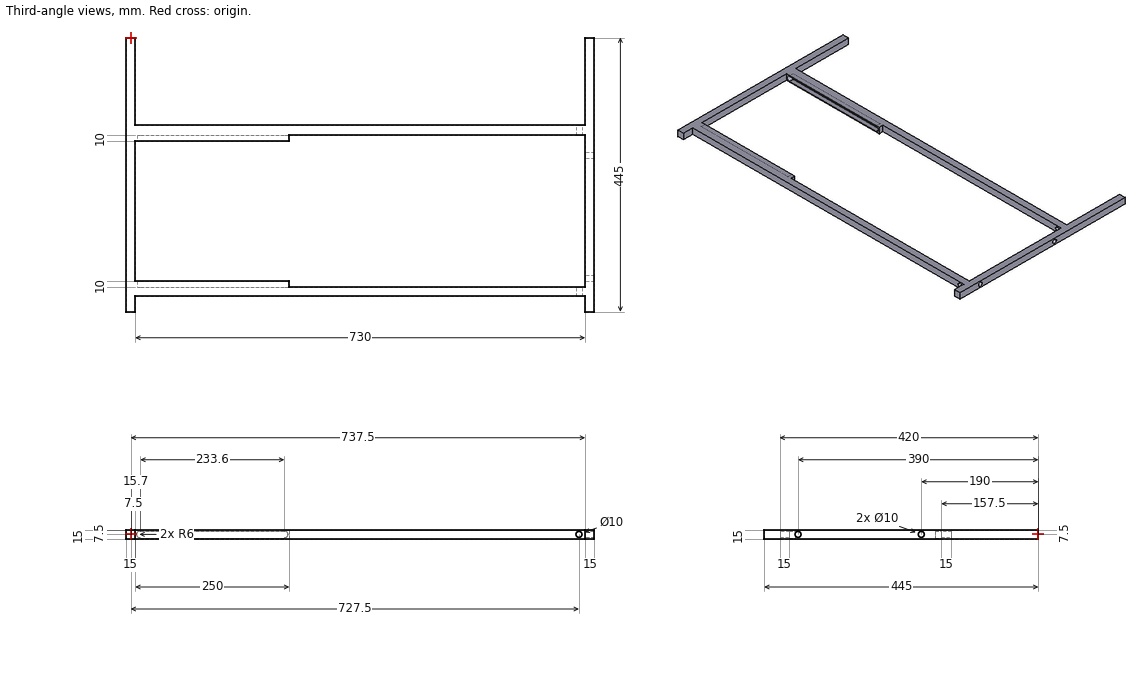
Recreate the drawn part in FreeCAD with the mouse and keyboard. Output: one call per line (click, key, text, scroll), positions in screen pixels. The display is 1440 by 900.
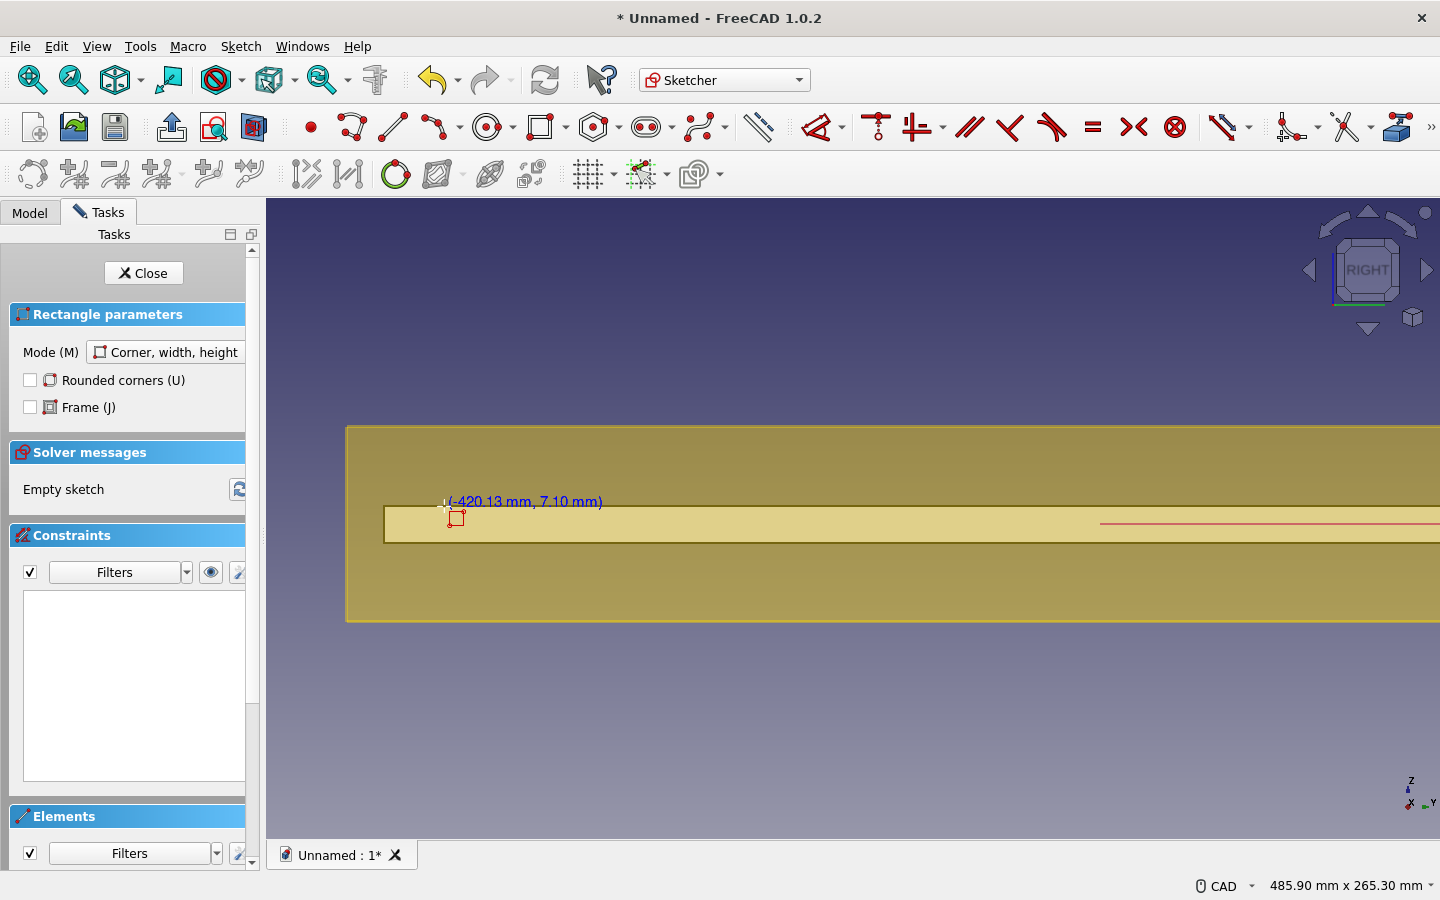
click(444, 506)
click(480, 543)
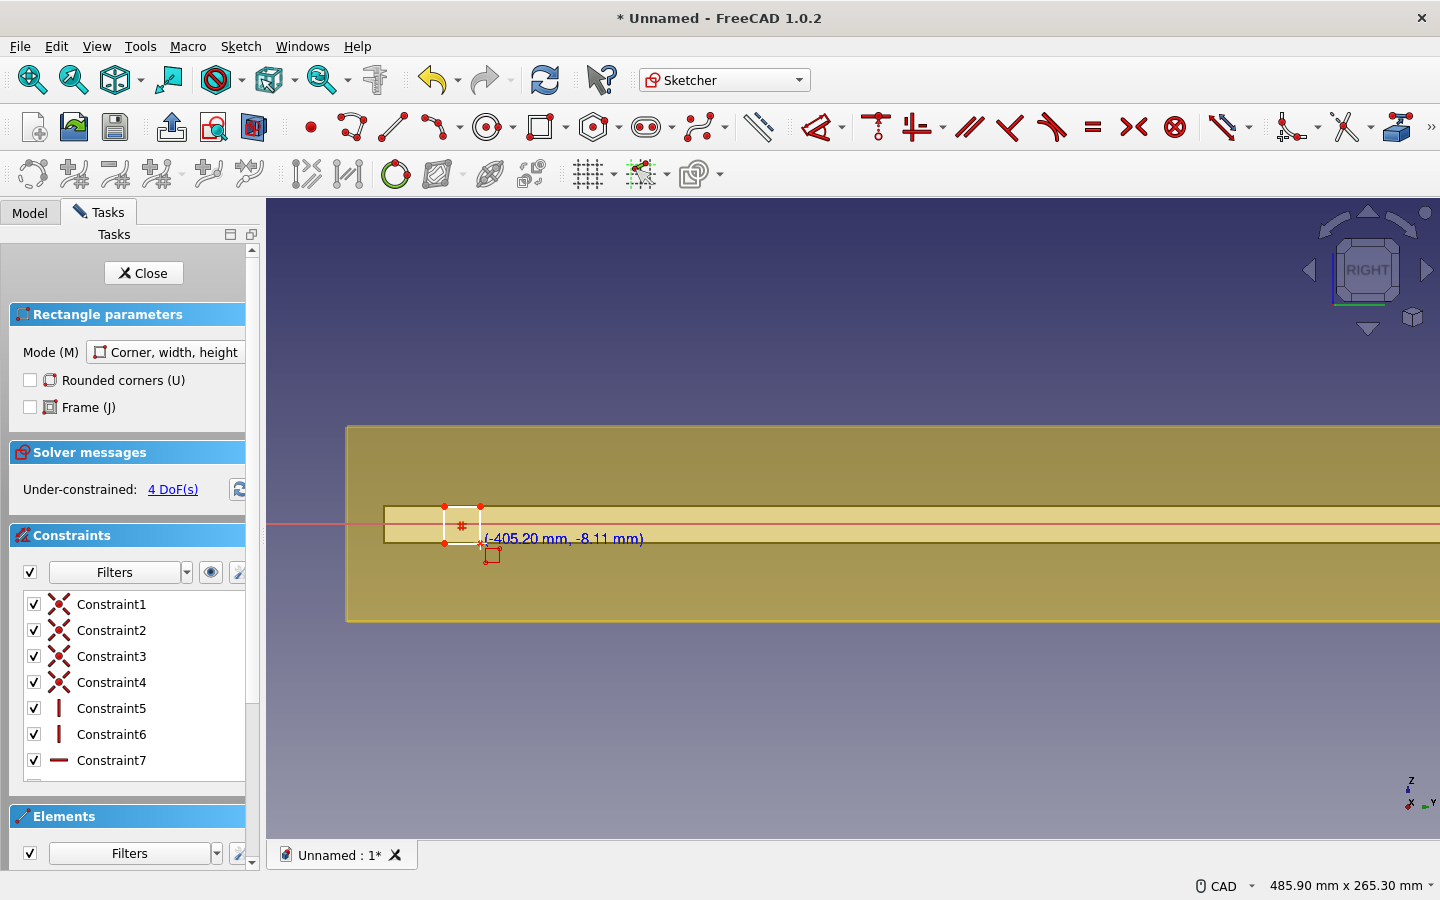
click(1078, 506)
click(1115, 543)
key(Escape)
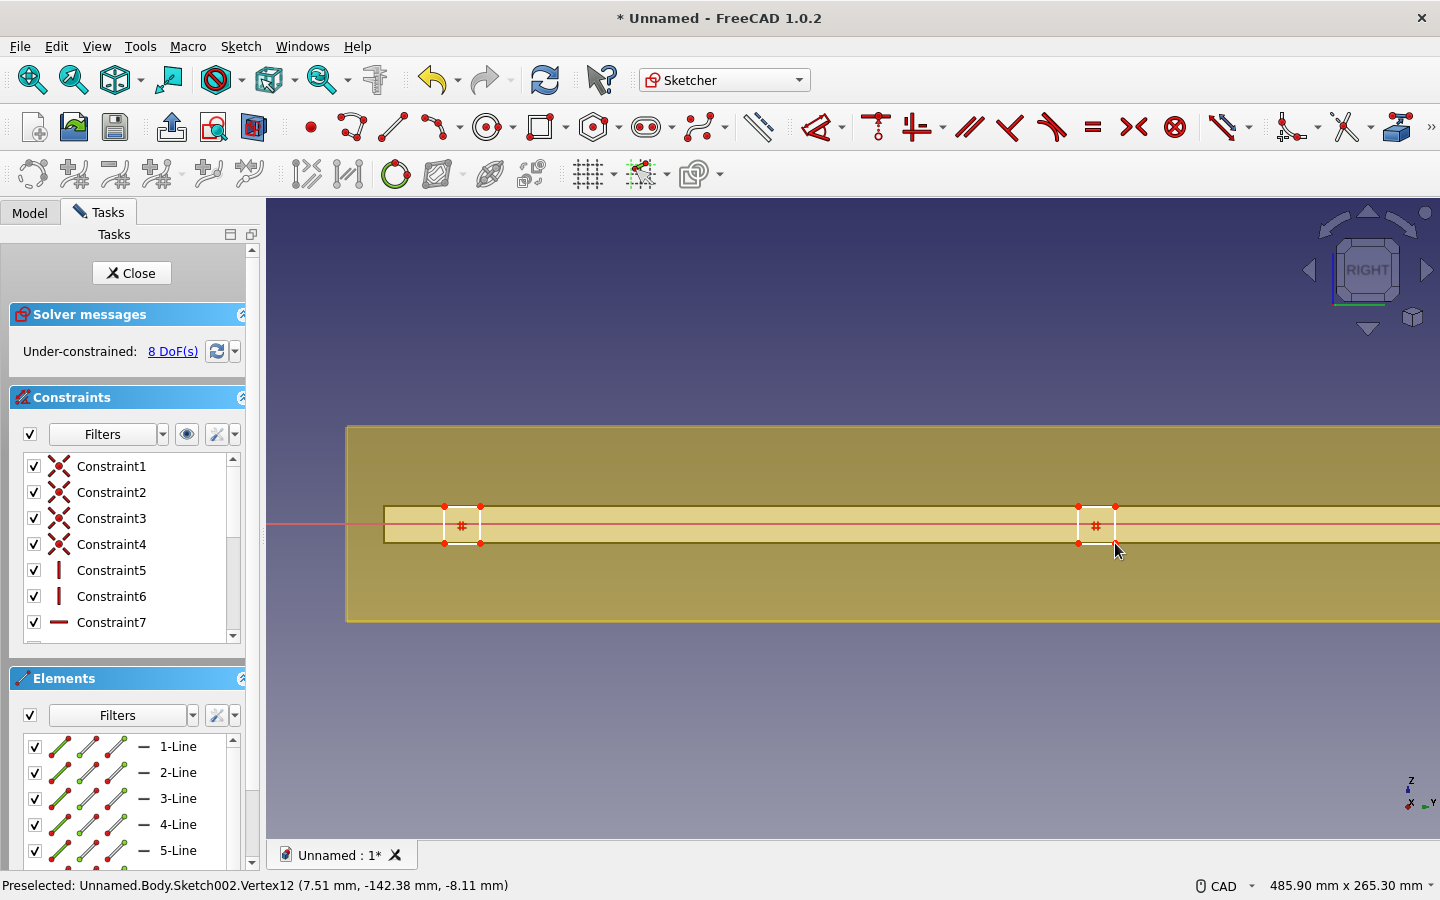
click(816, 128)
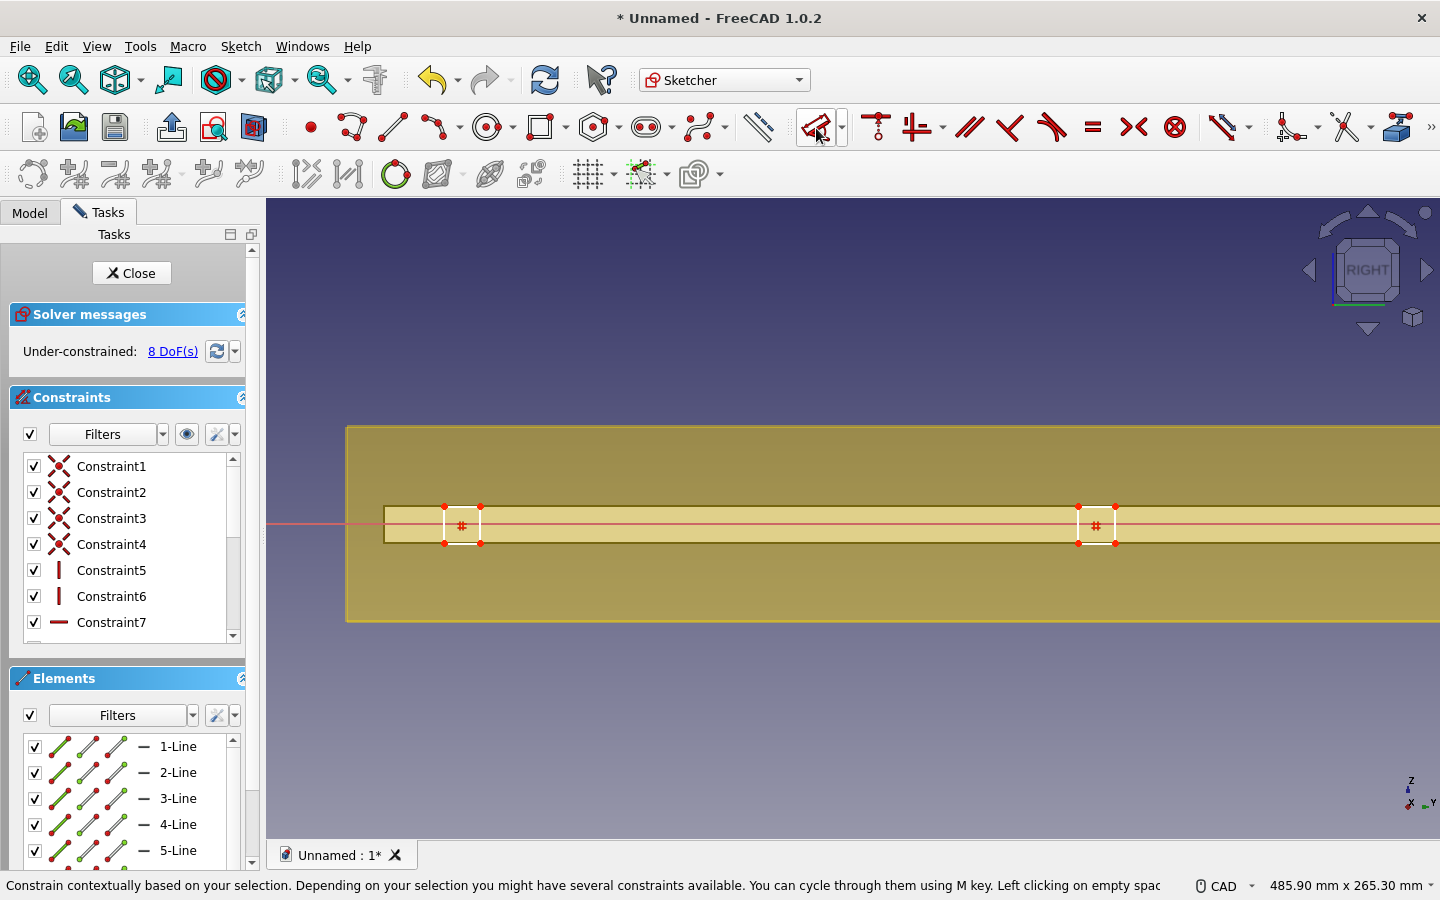
click(444, 522)
click(410, 538)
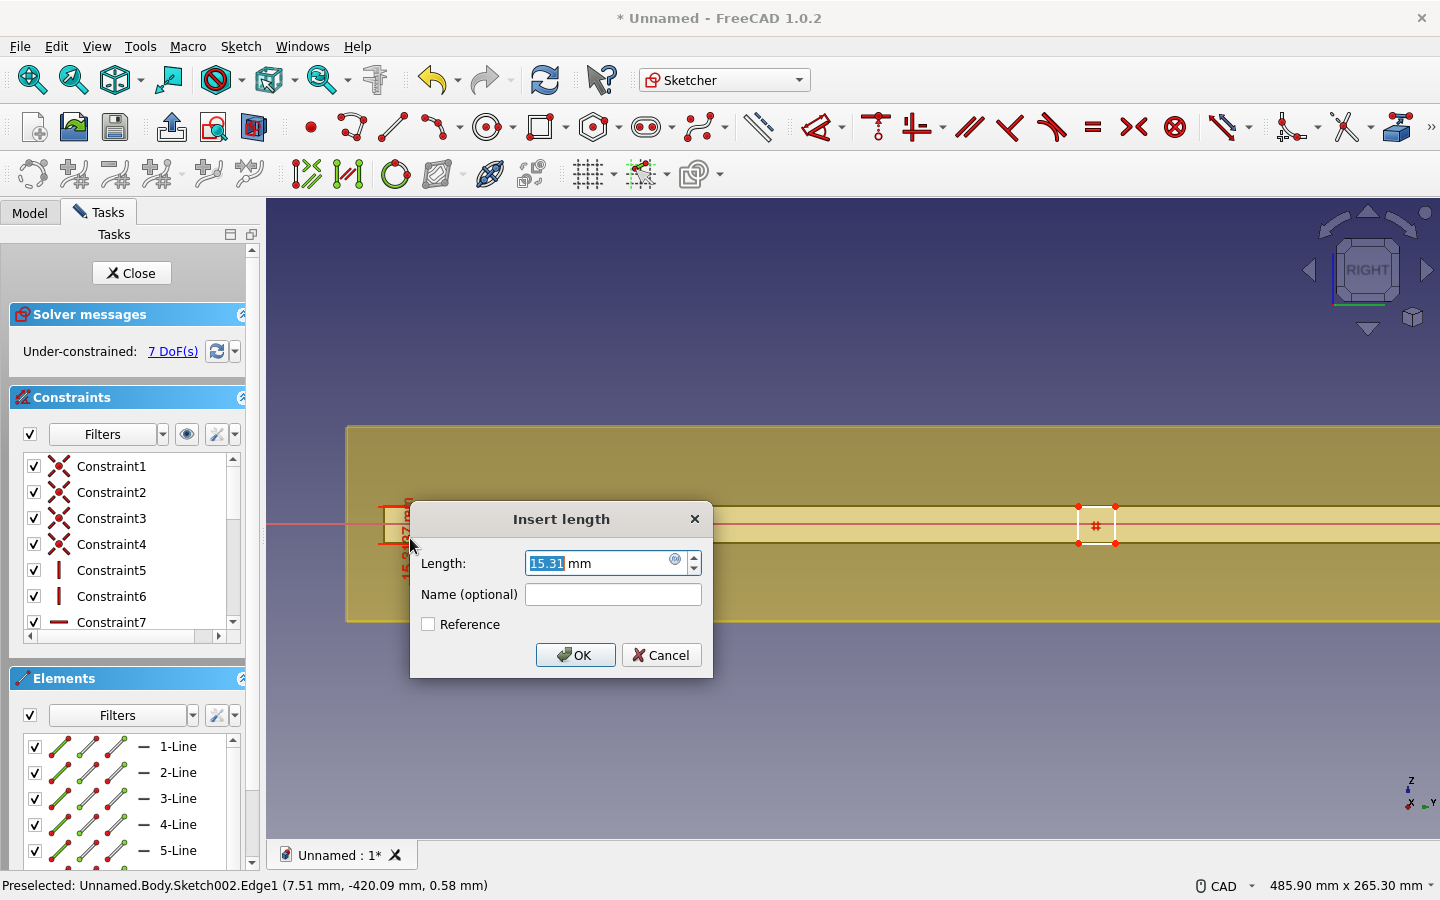
text(15)
key(Return)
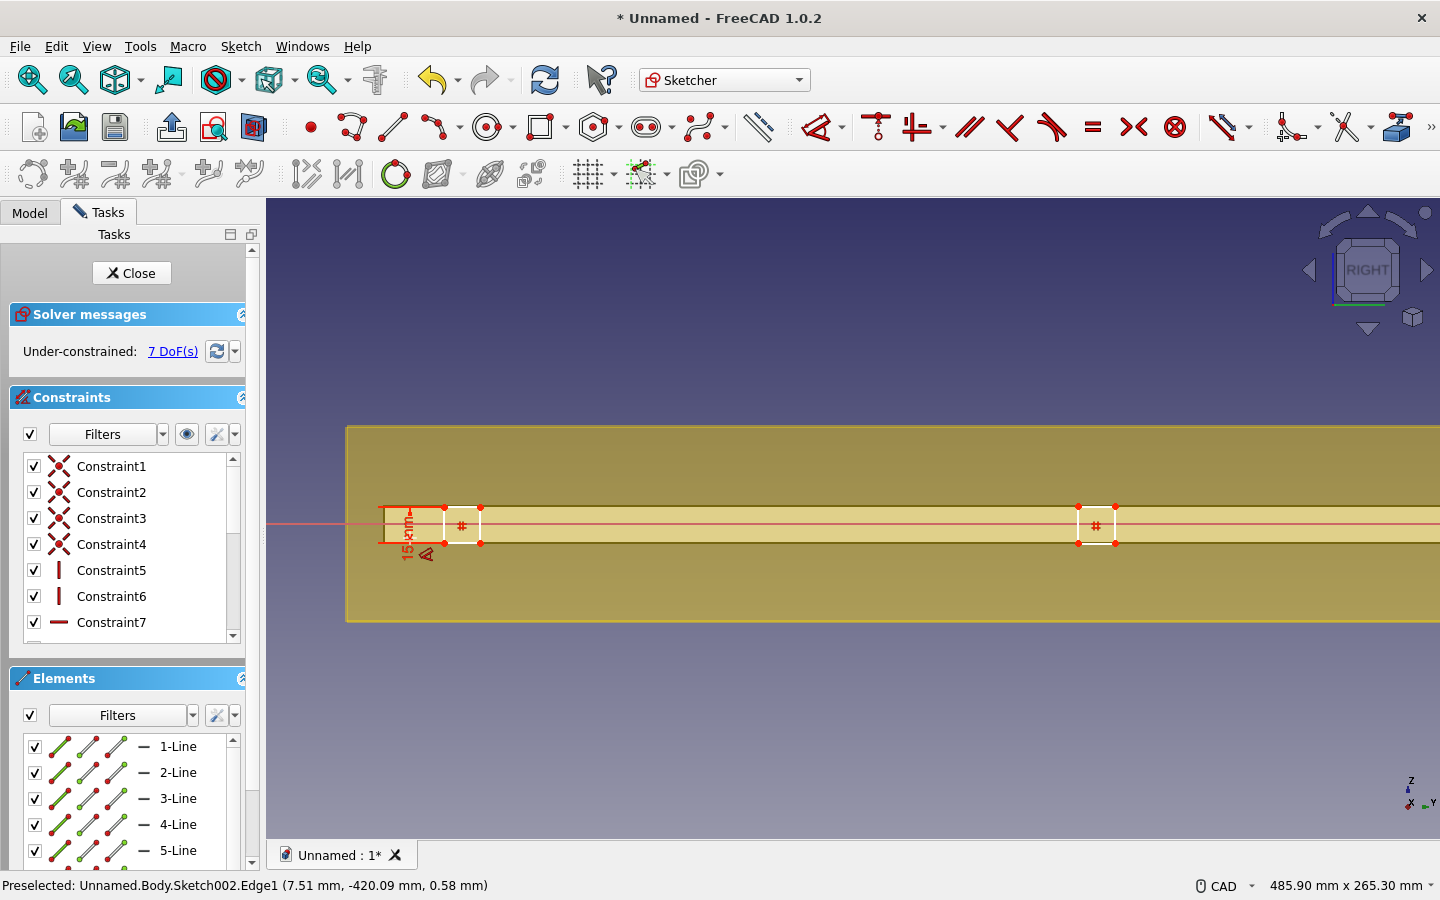
scroll(455, 543, up, 2)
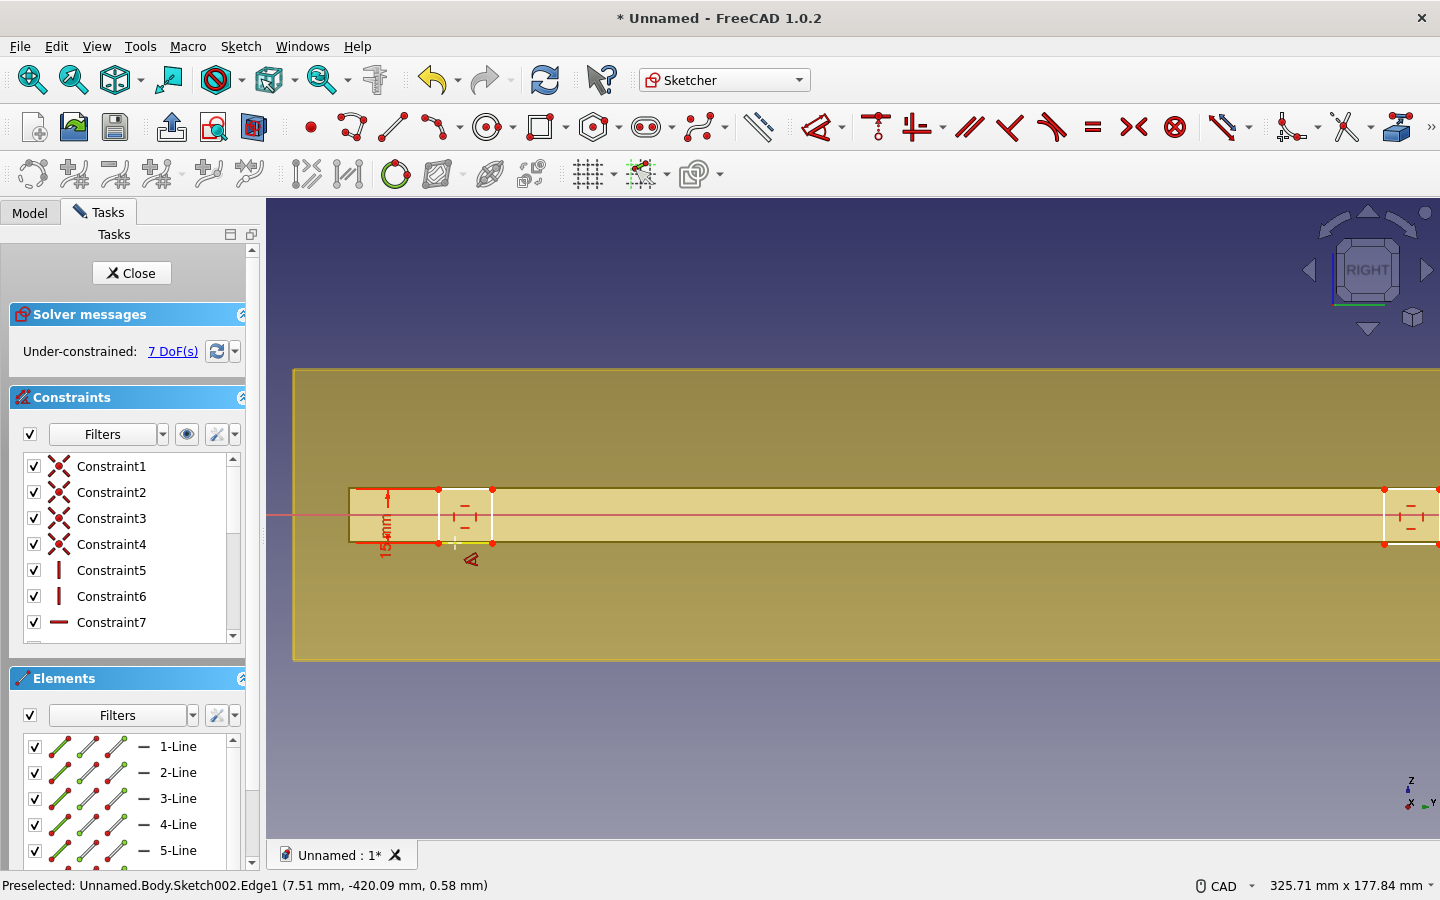
click(455, 543)
click(465, 577)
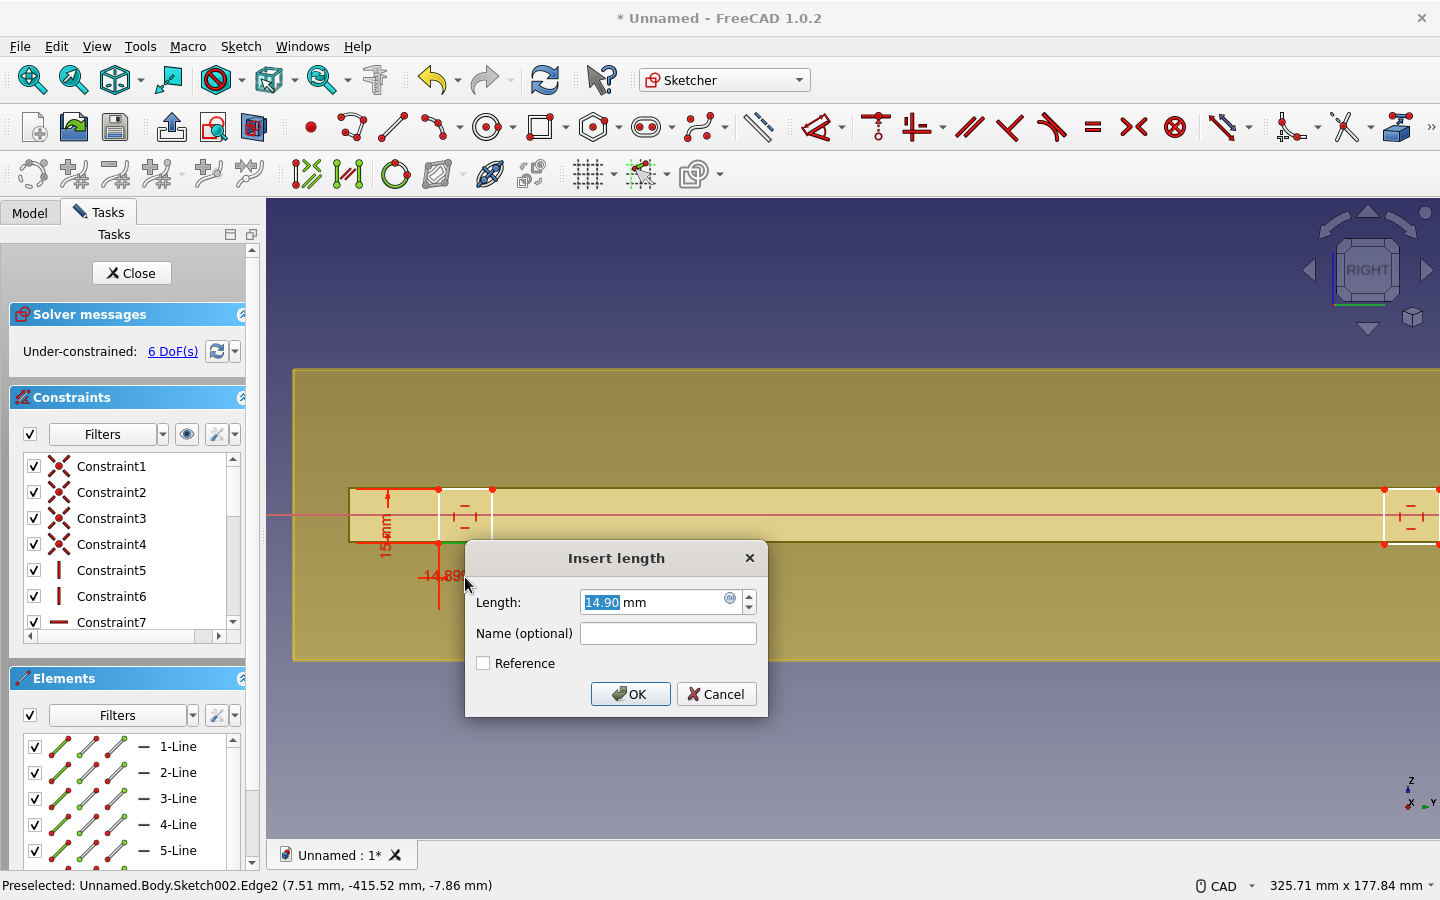
text(15)
key(Return)